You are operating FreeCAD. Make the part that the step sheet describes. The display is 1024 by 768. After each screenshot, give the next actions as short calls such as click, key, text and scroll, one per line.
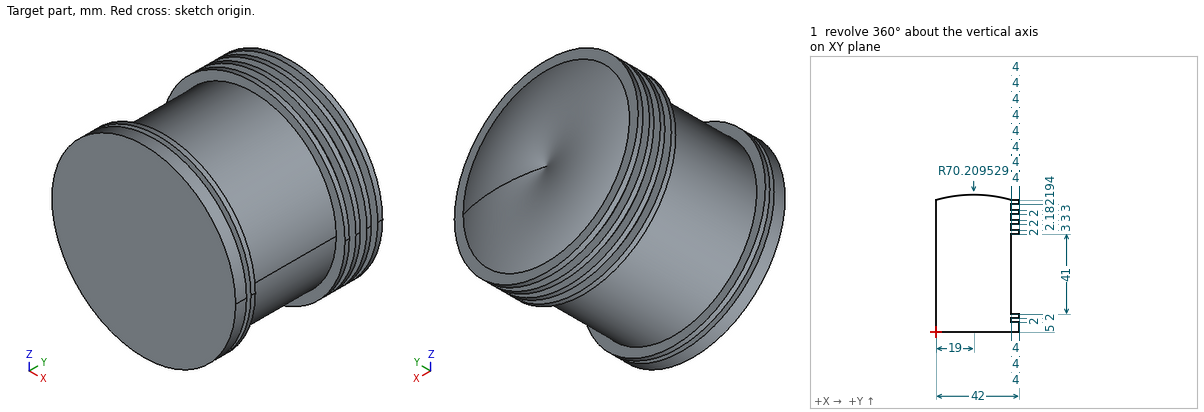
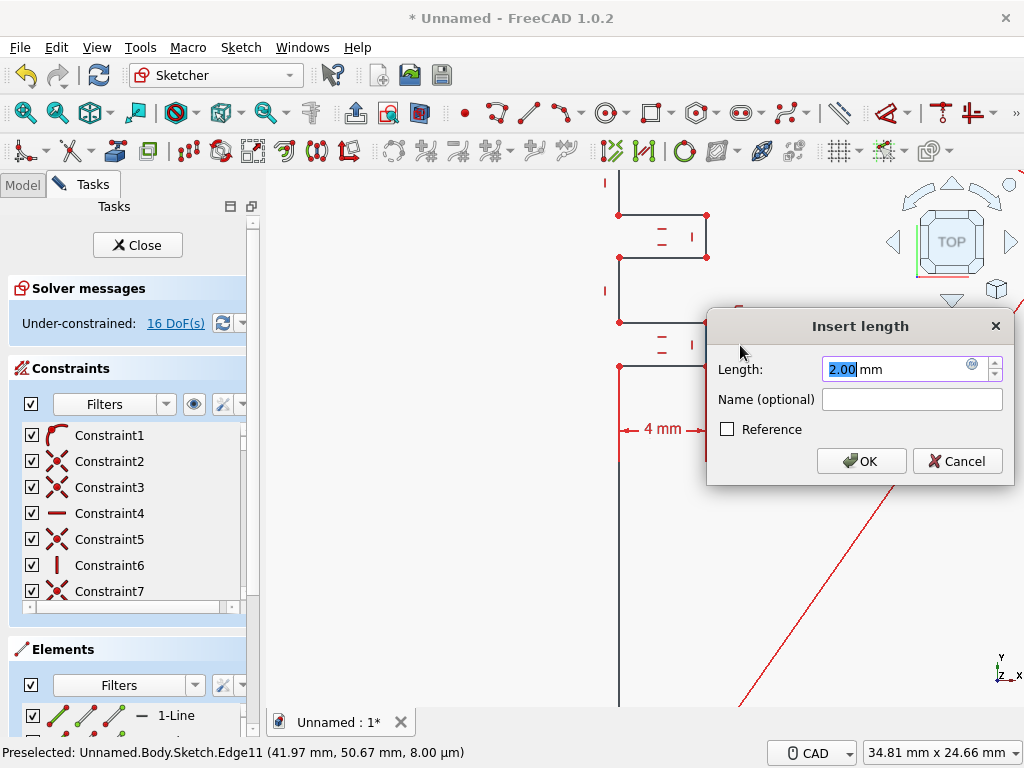
text(2)
key(Return)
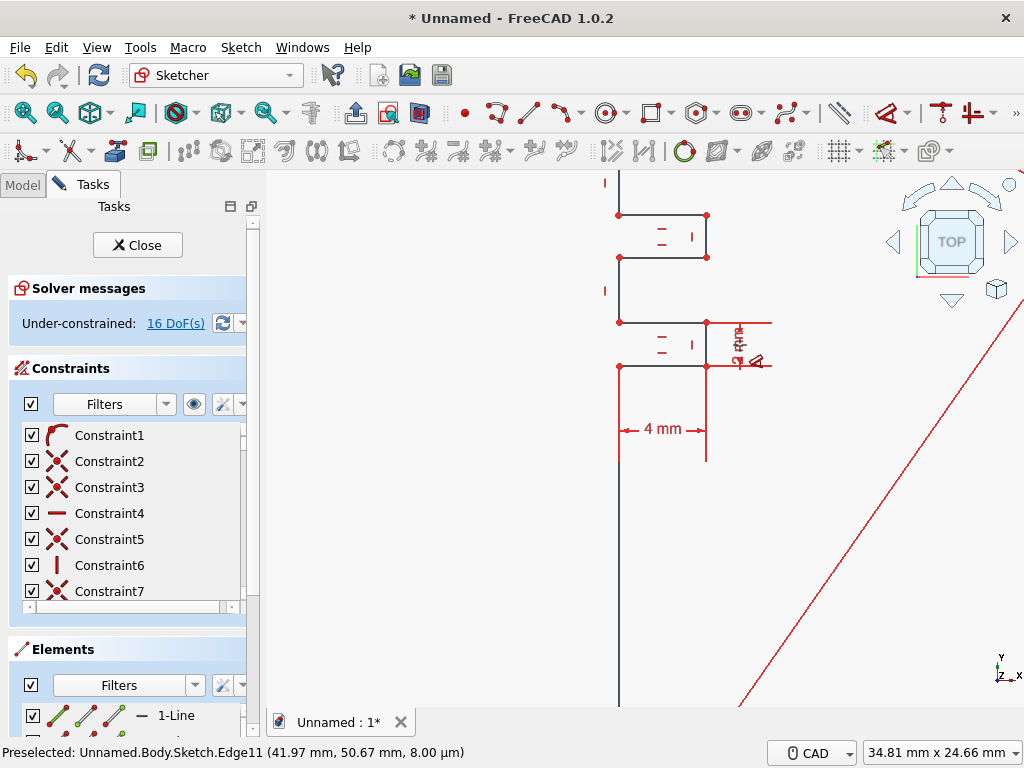
click(680, 323)
click(663, 289)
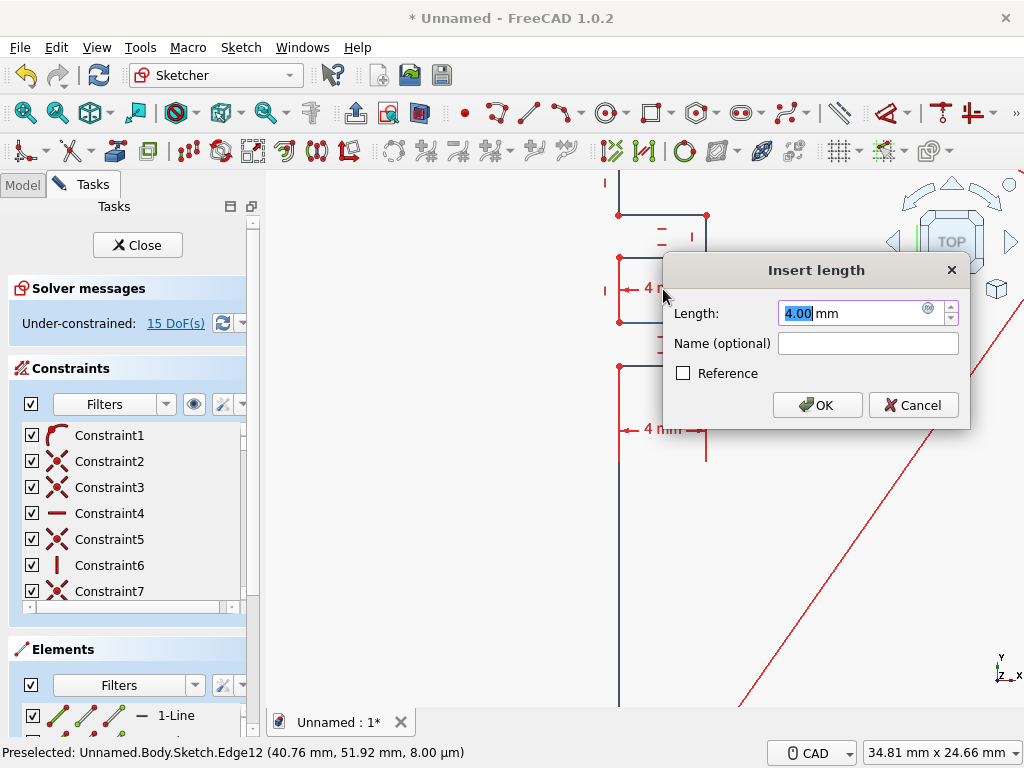
text(4)
key(Return)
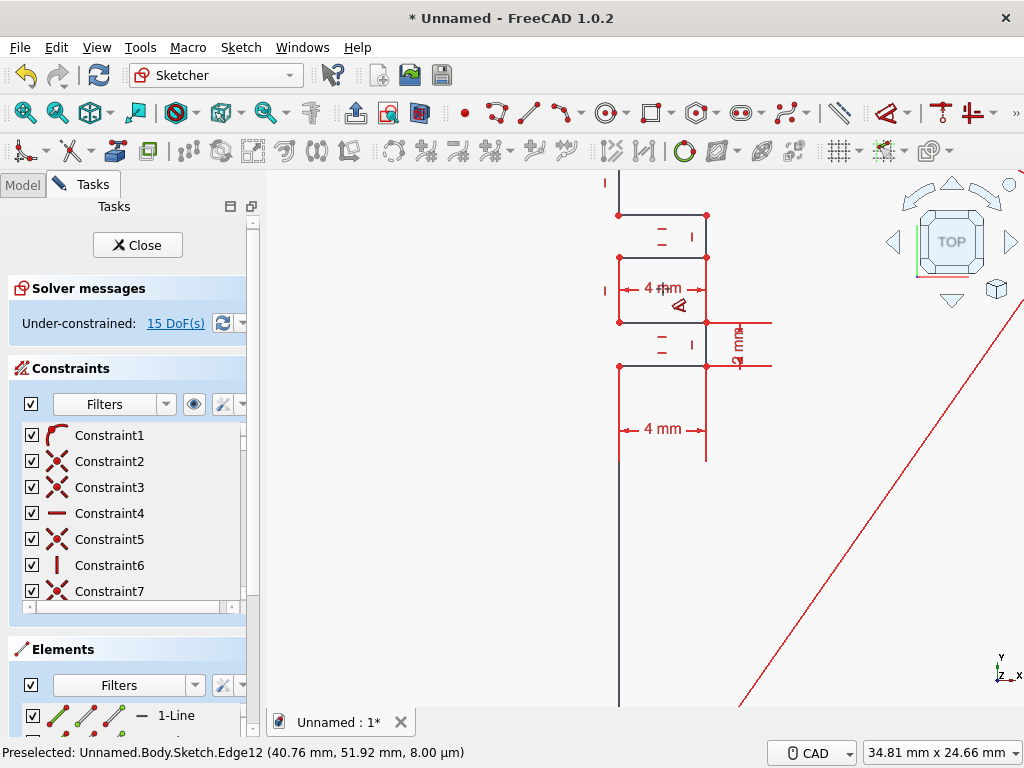
click(619, 303)
click(585, 290)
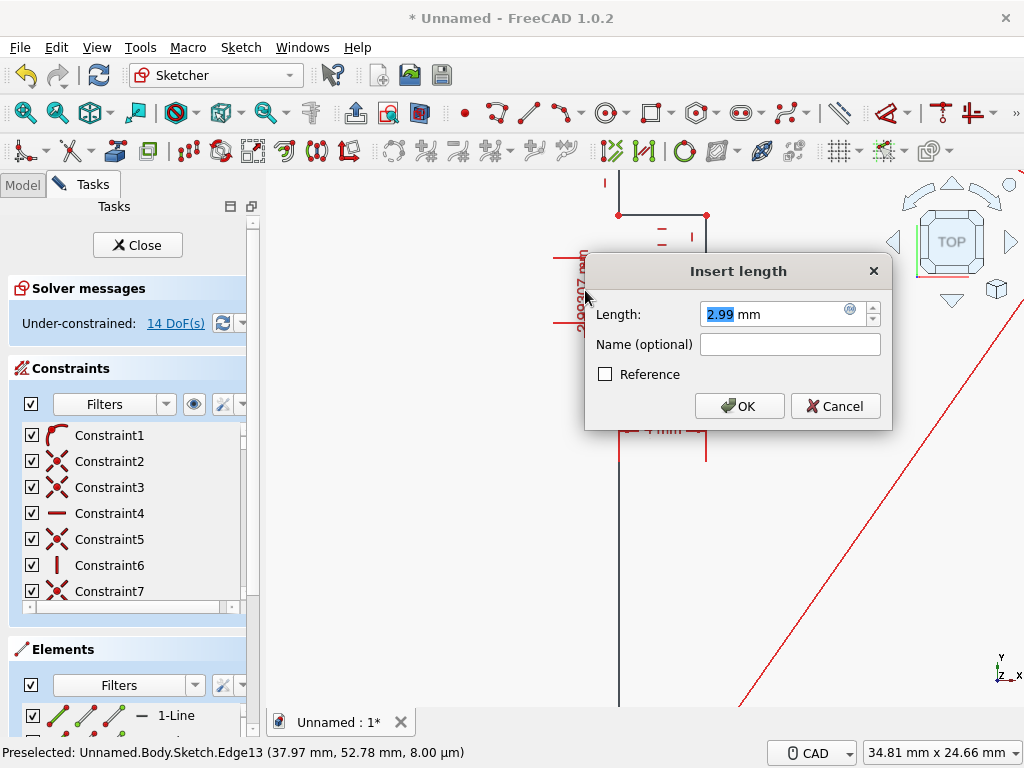
text(3)
key(Return)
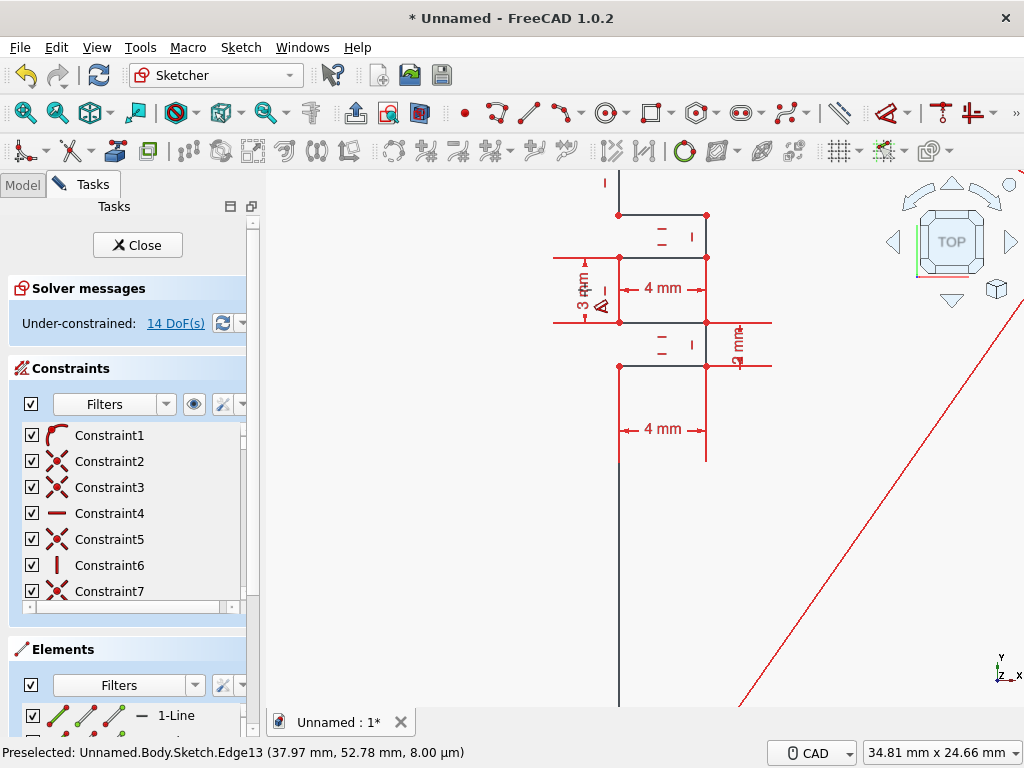
click(645, 258)
click(663, 200)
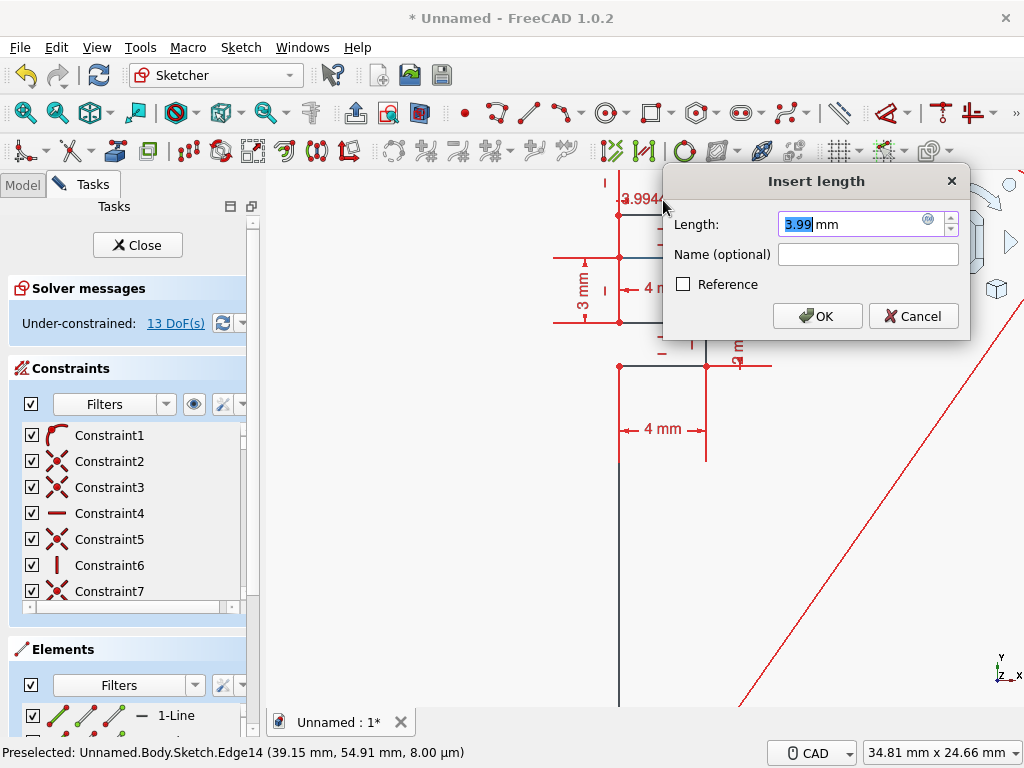
text(4)
key(Return)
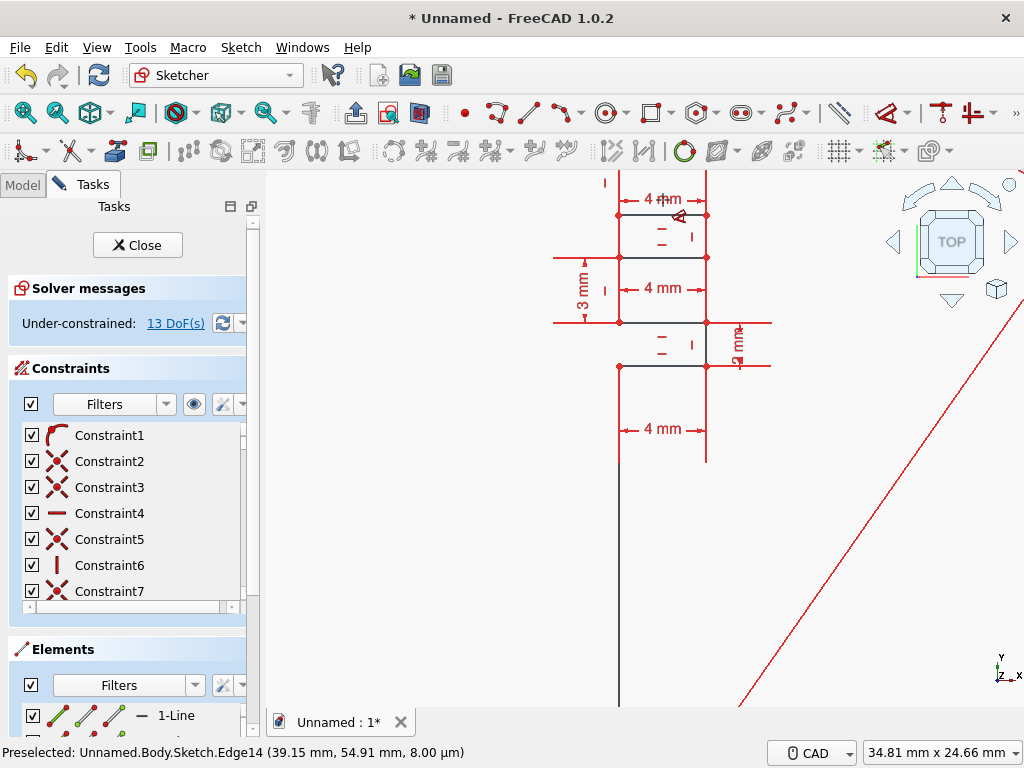
click(706, 245)
click(740, 236)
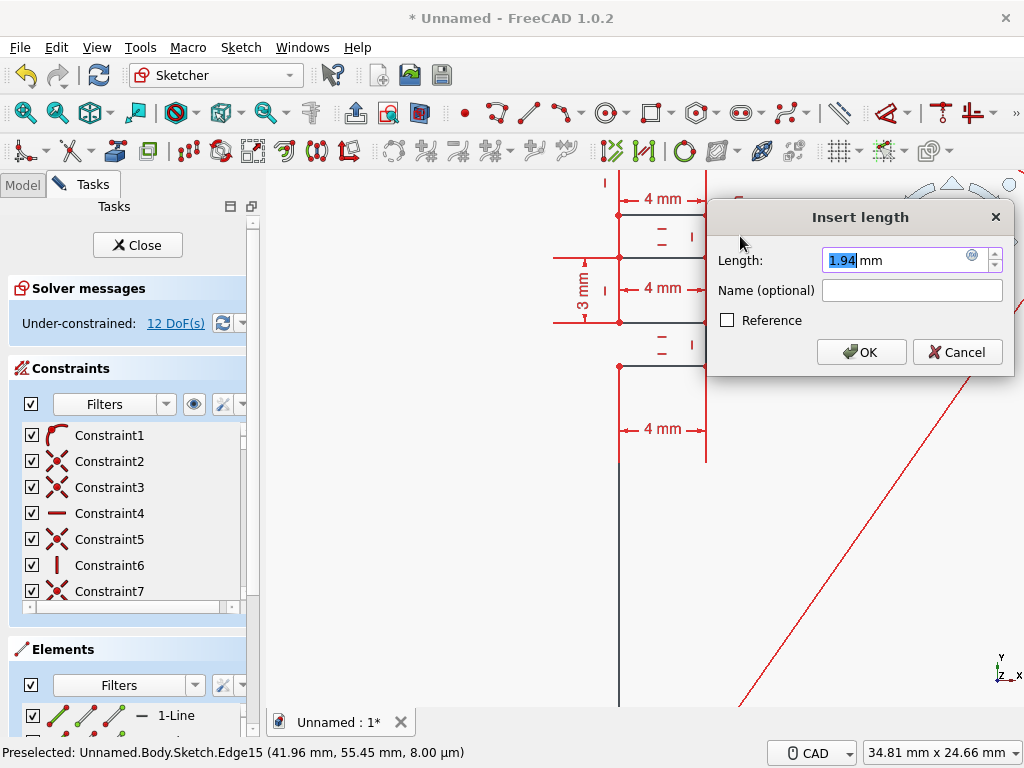
text(2)
key(Return)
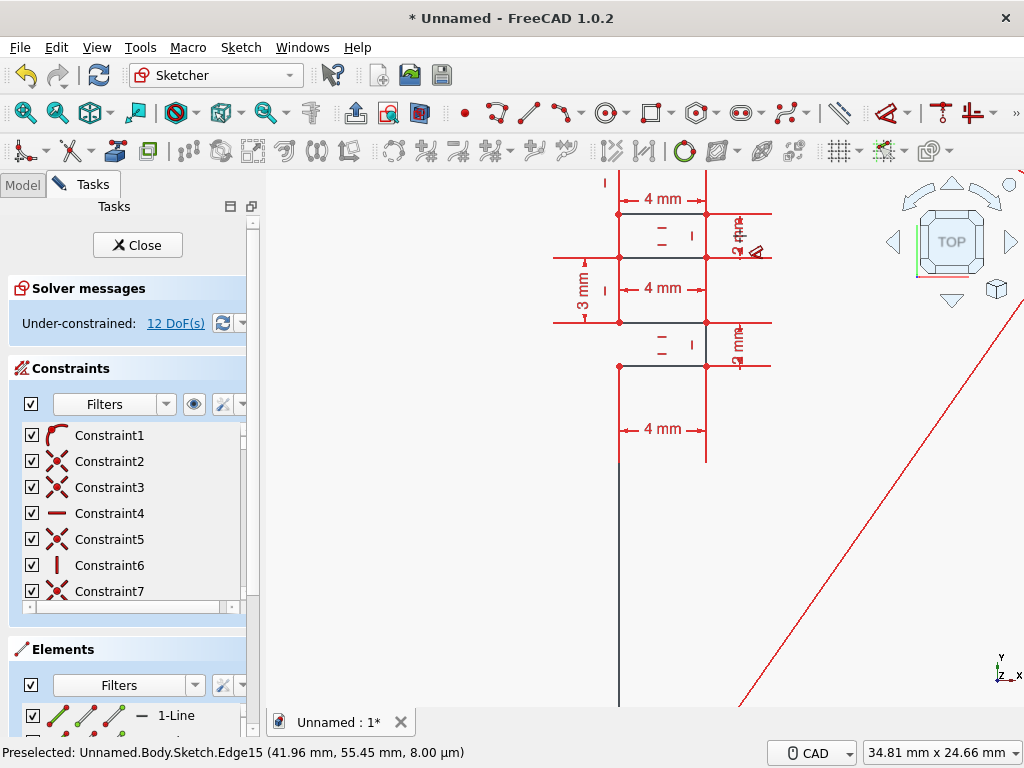
click(680, 214)
click(663, 344)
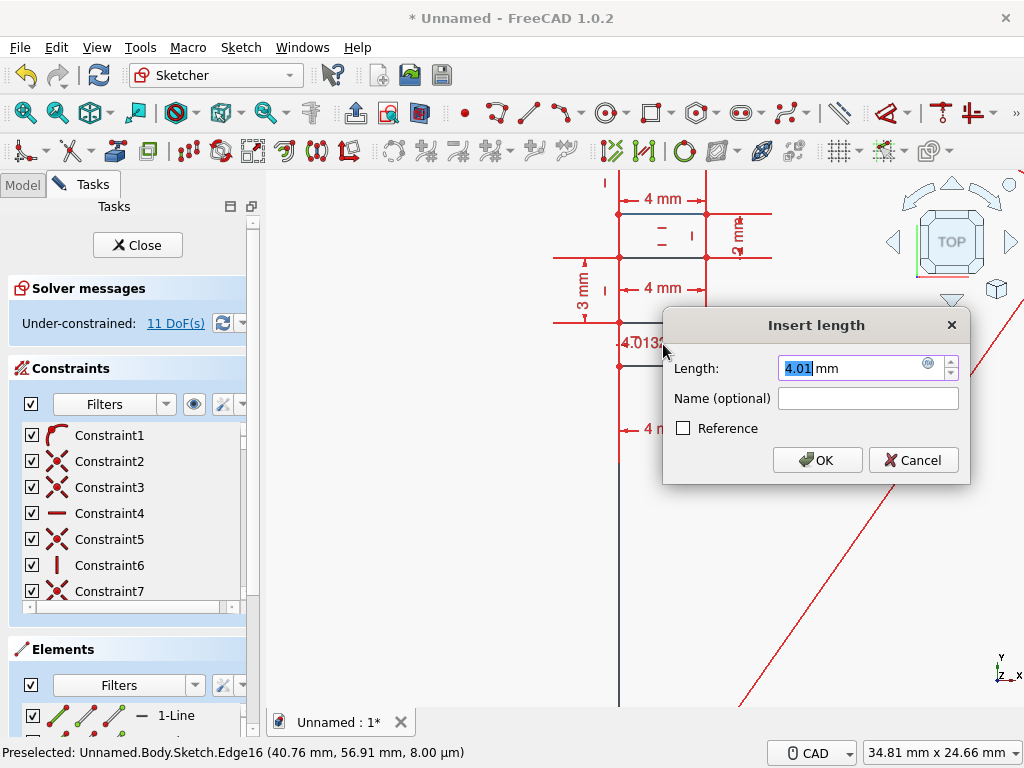
text(4)
key(Return)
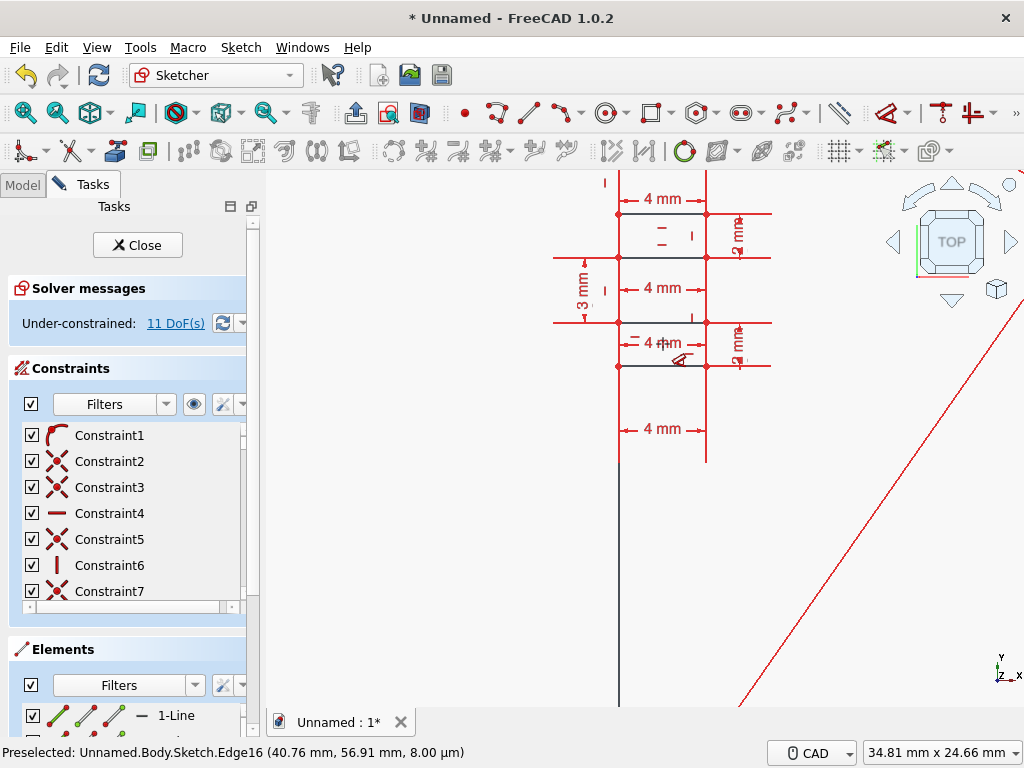
click(619, 201)
click(585, 206)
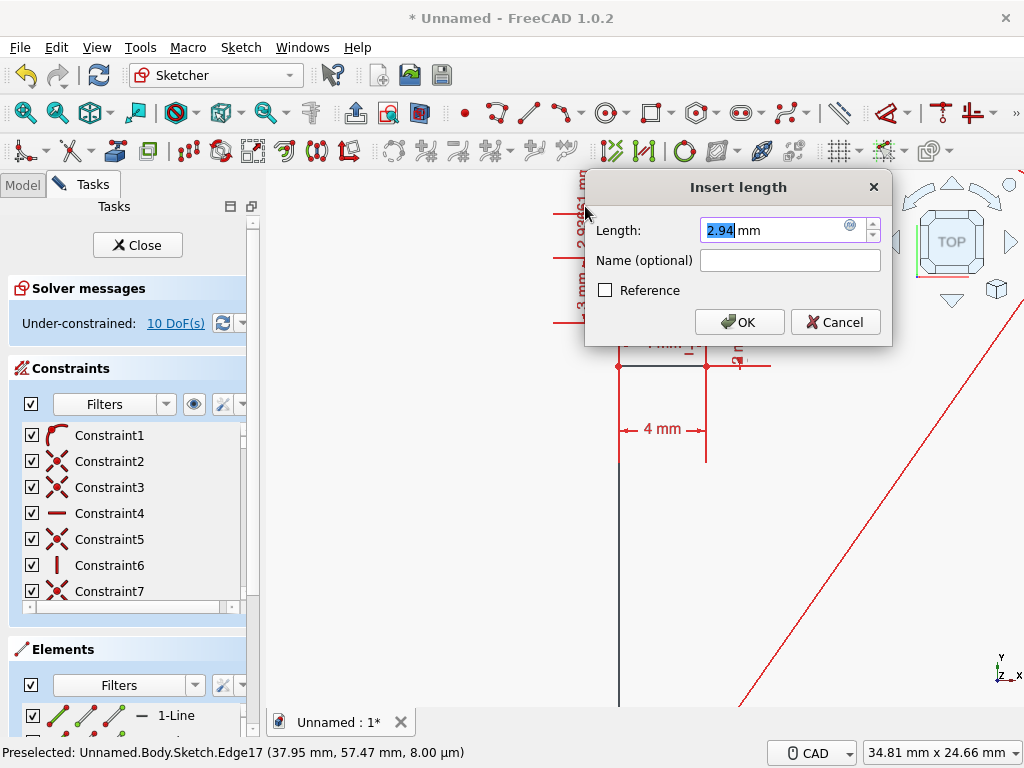
text(3)
key(Return)